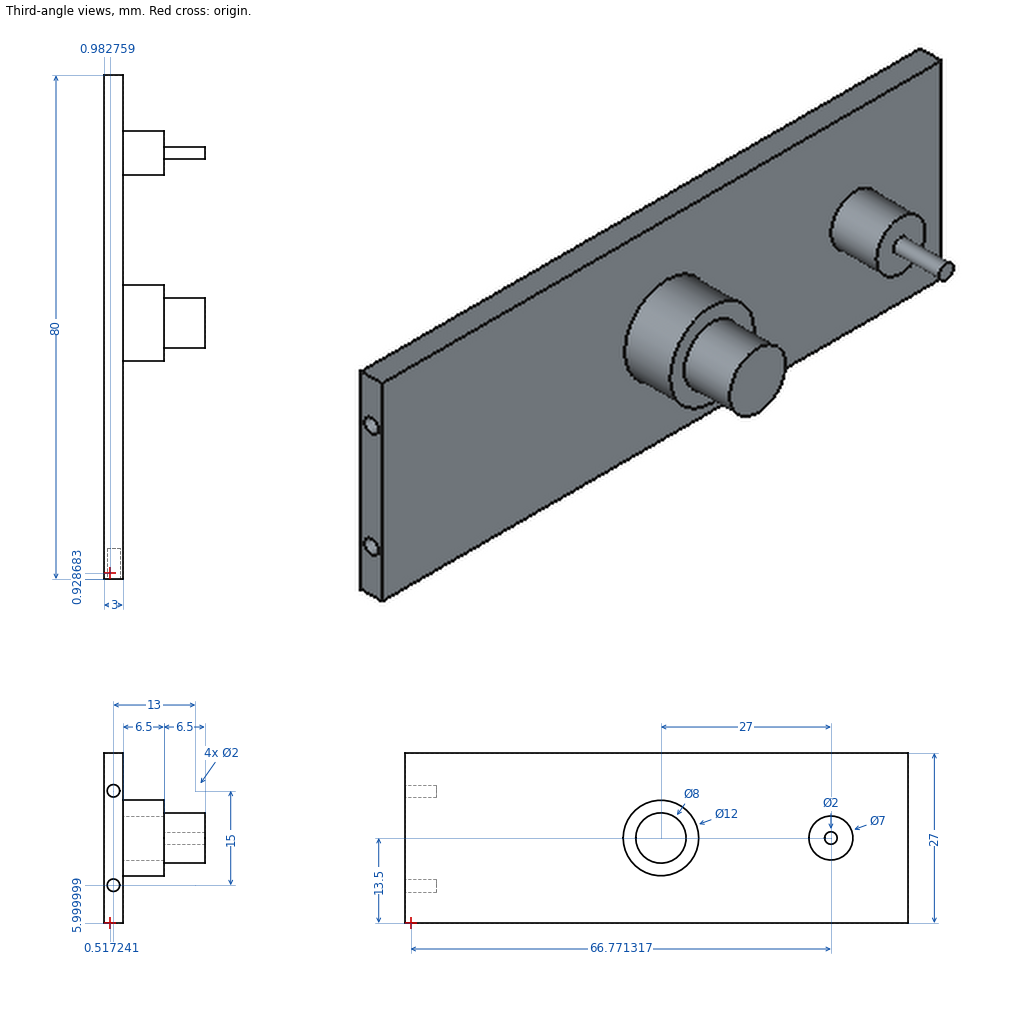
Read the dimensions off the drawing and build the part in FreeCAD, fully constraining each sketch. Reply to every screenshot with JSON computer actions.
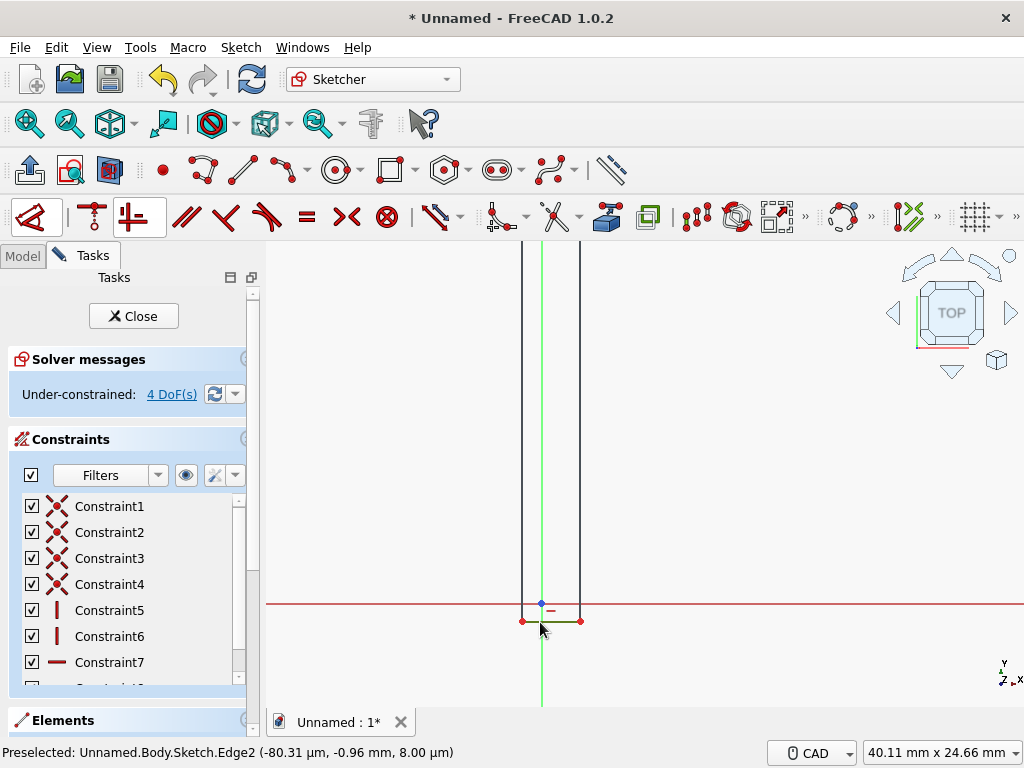
{"action": "key", "text": "l"}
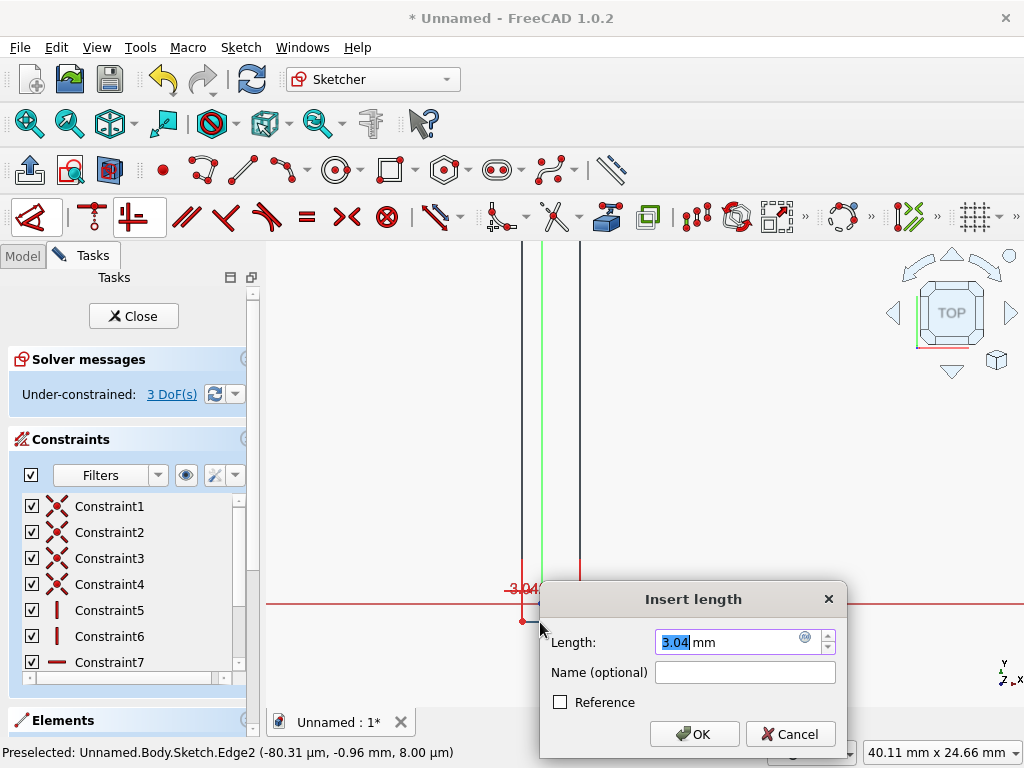
{"action": "type", "text": "3"}
{"action": "key", "text": "Return"}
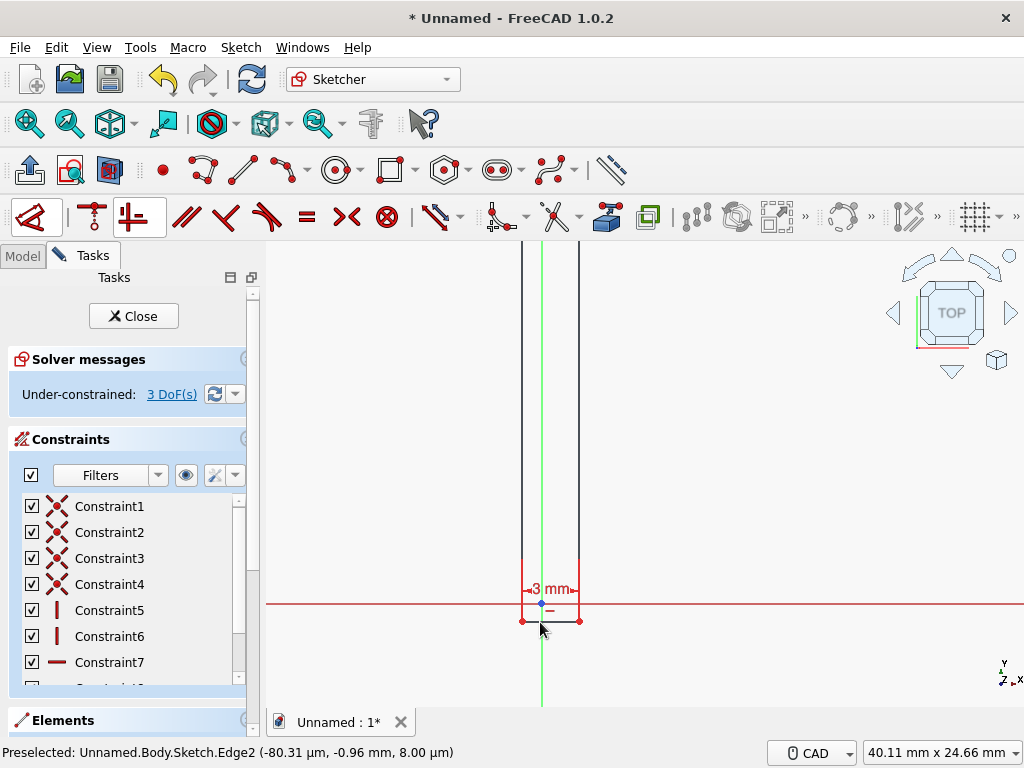
{"action": "left_click", "coordinate": [523, 320]}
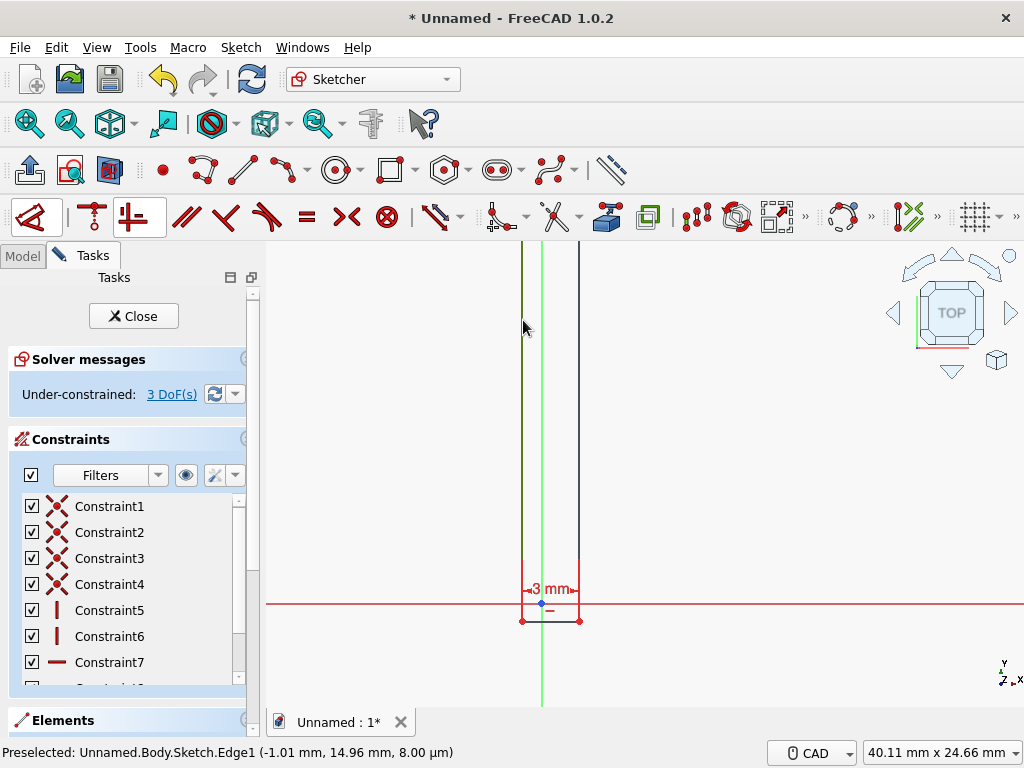
{"action": "key", "text": "i"}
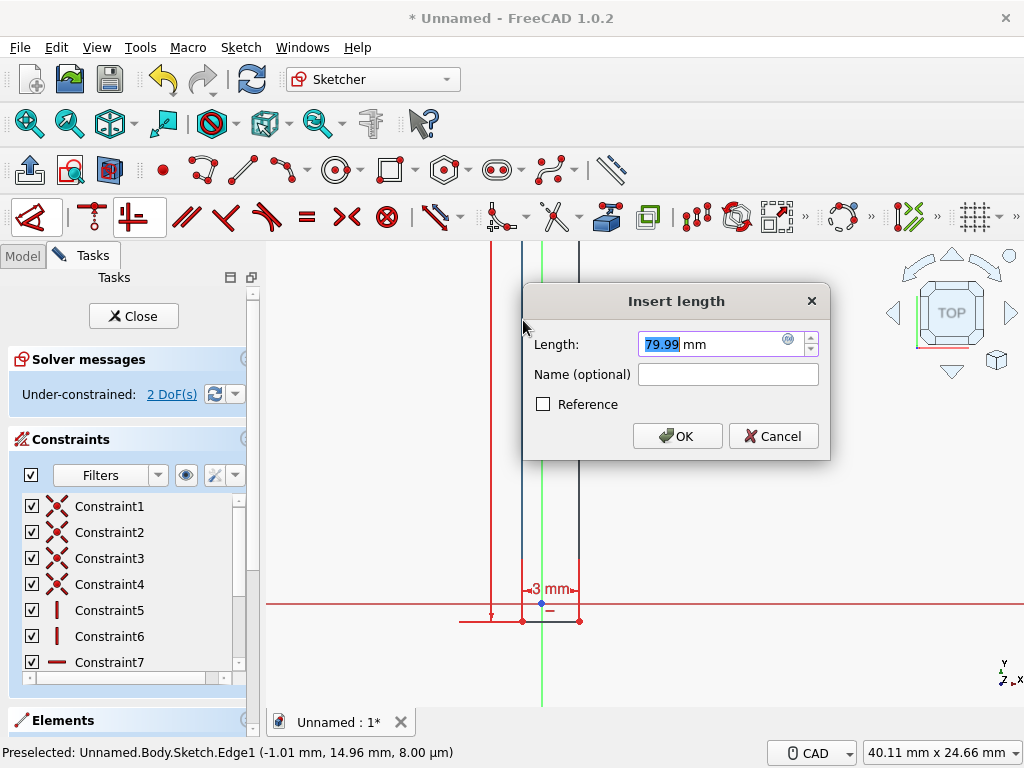
{"action": "type", "text": "80"}
{"action": "key", "text": "Return"}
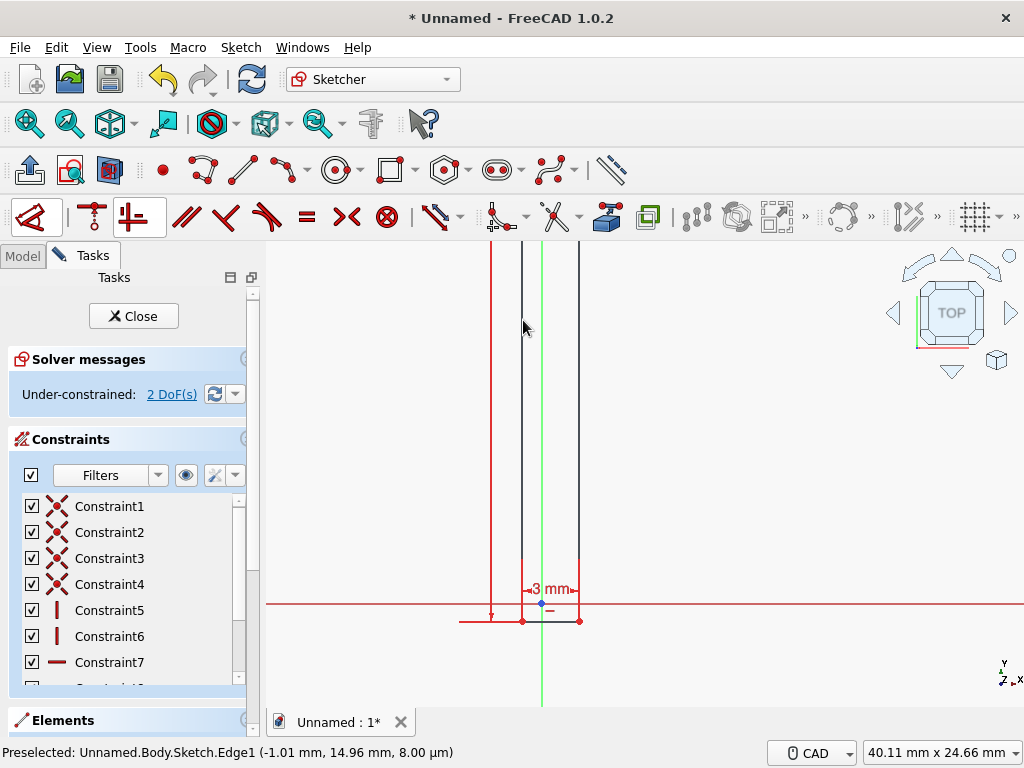
{"action": "scroll", "coordinate": [583, 628], "scroll_direction": "down", "scroll_amount": 8}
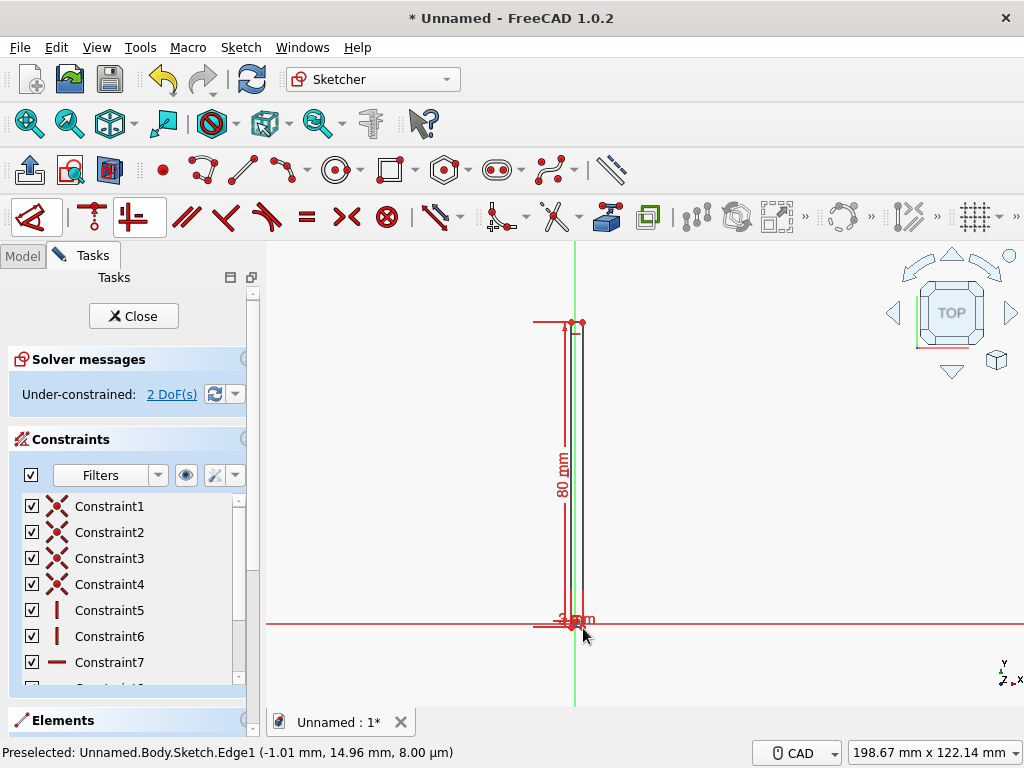
{"action": "scroll", "coordinate": [571, 322], "scroll_direction": "up", "scroll_amount": 12}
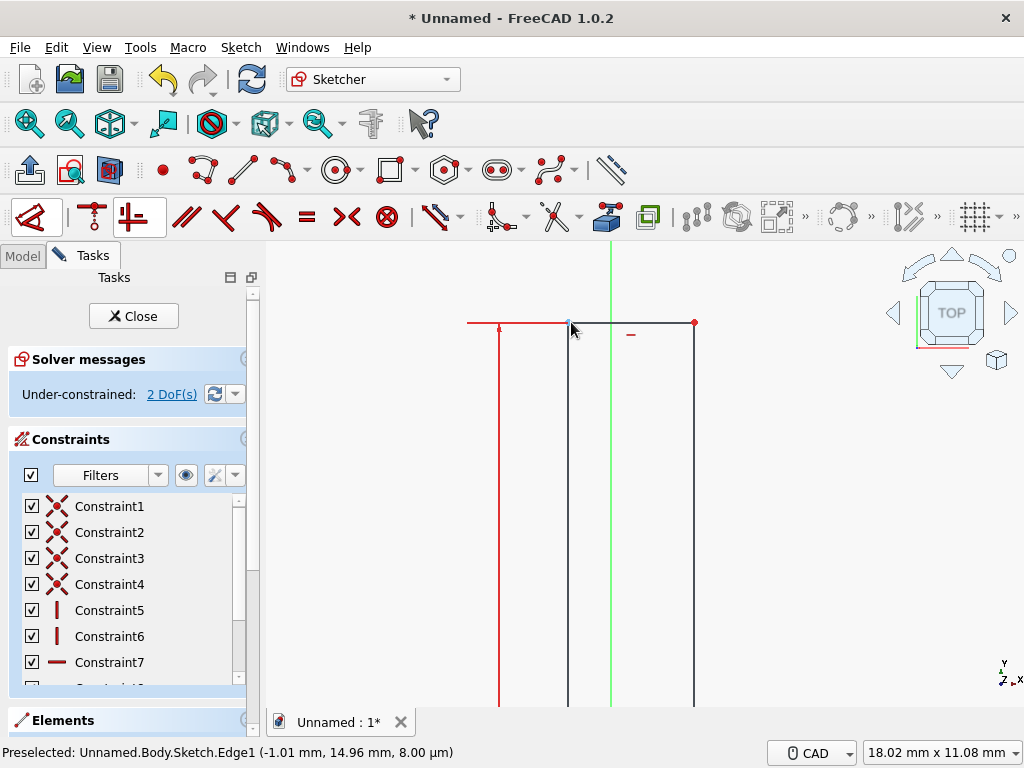
{"action": "left_click", "coordinate": [568, 323]}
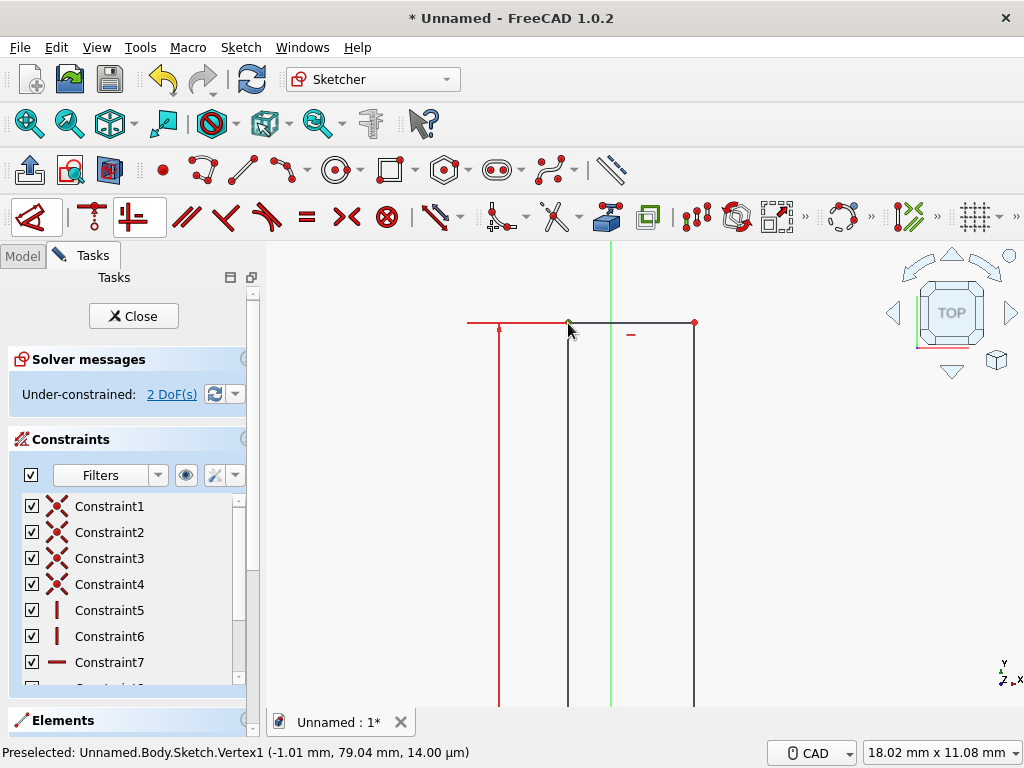
{"action": "key", "text": "l"}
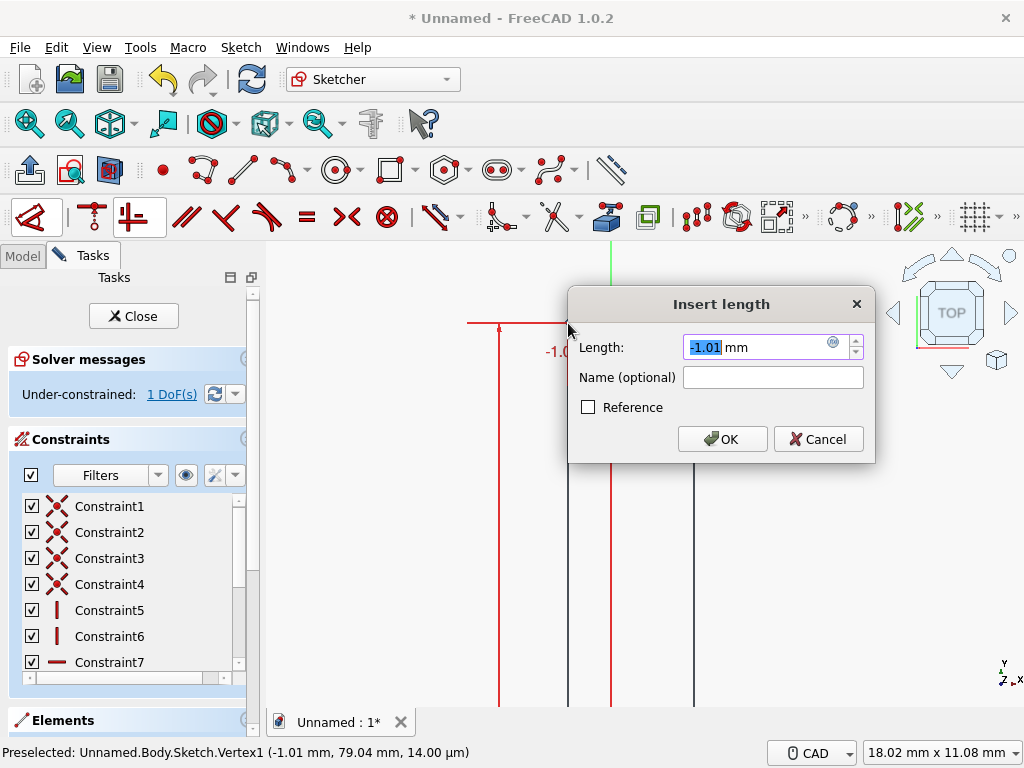
{"action": "type", "text": "-0.982759"}
{"action": "key", "text": "Return"}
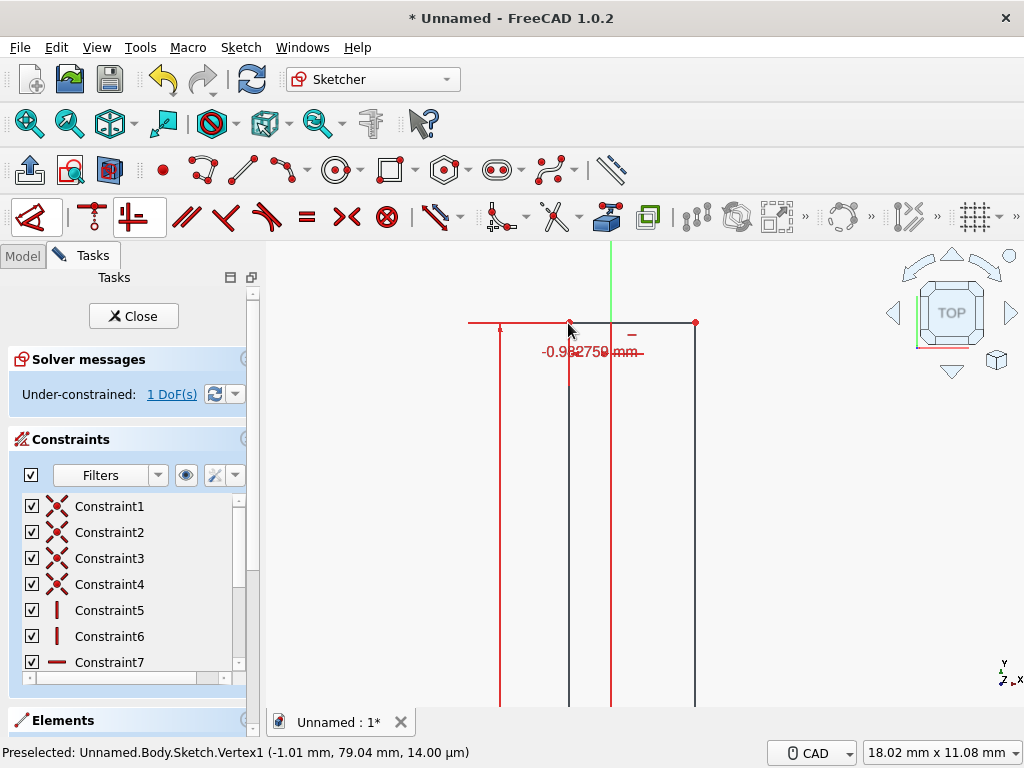
{"action": "scroll", "coordinate": [571, 321], "scroll_direction": "down", "scroll_amount": 12}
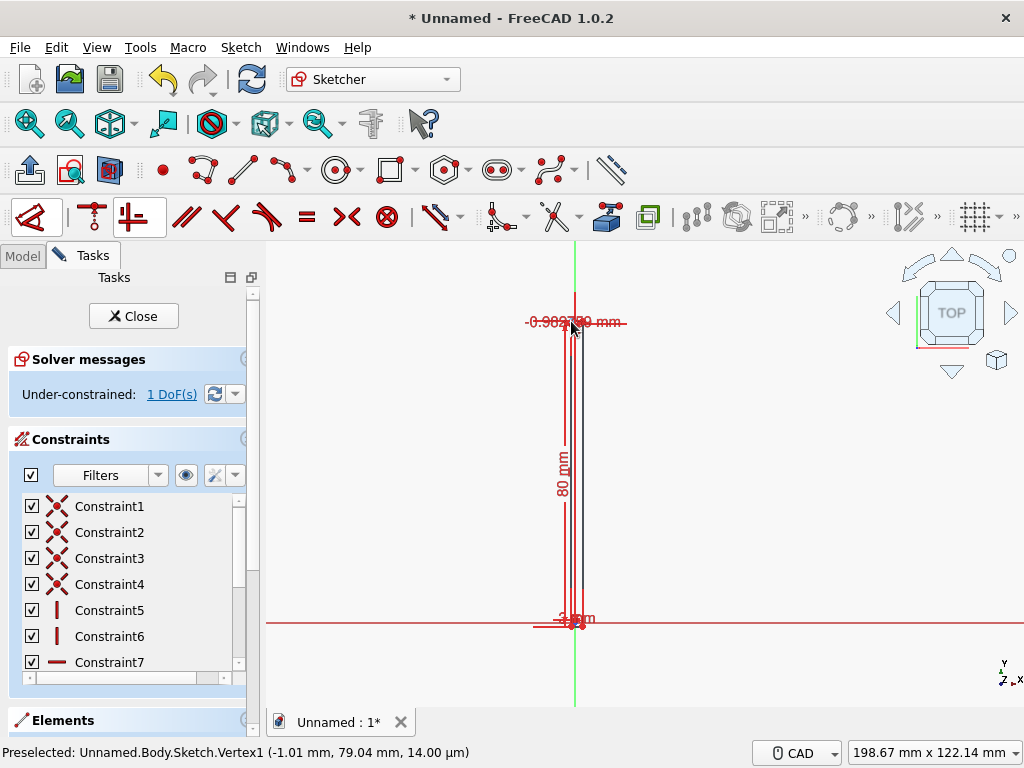
{"action": "scroll", "coordinate": [571, 627], "scroll_direction": "up", "scroll_amount": 13}